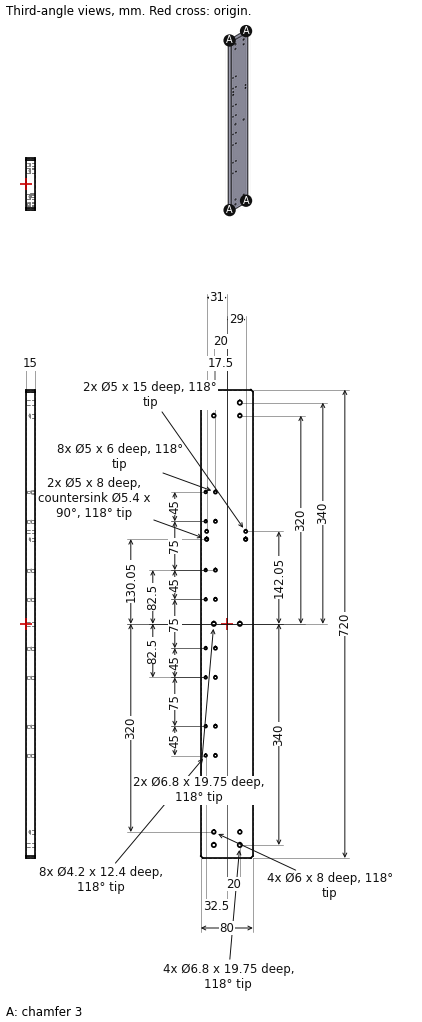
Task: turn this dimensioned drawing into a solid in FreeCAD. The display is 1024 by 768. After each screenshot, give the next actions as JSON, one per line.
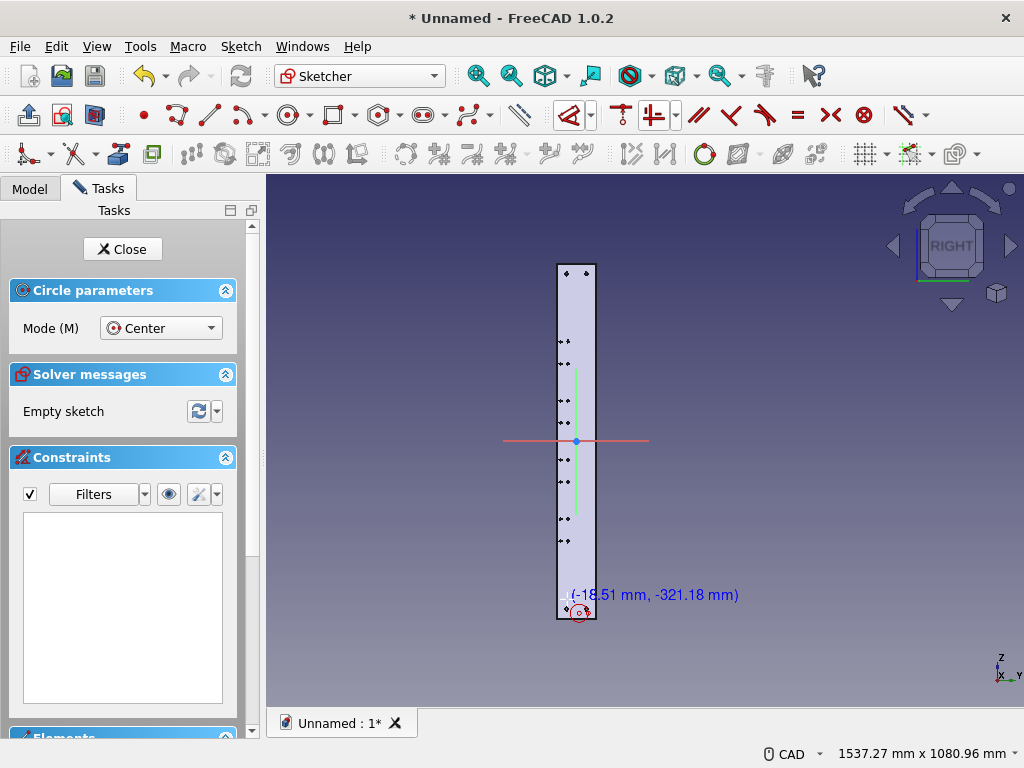
{"action": "scroll", "coordinate": [567, 599], "scroll_direction": "up", "scroll_amount": 3}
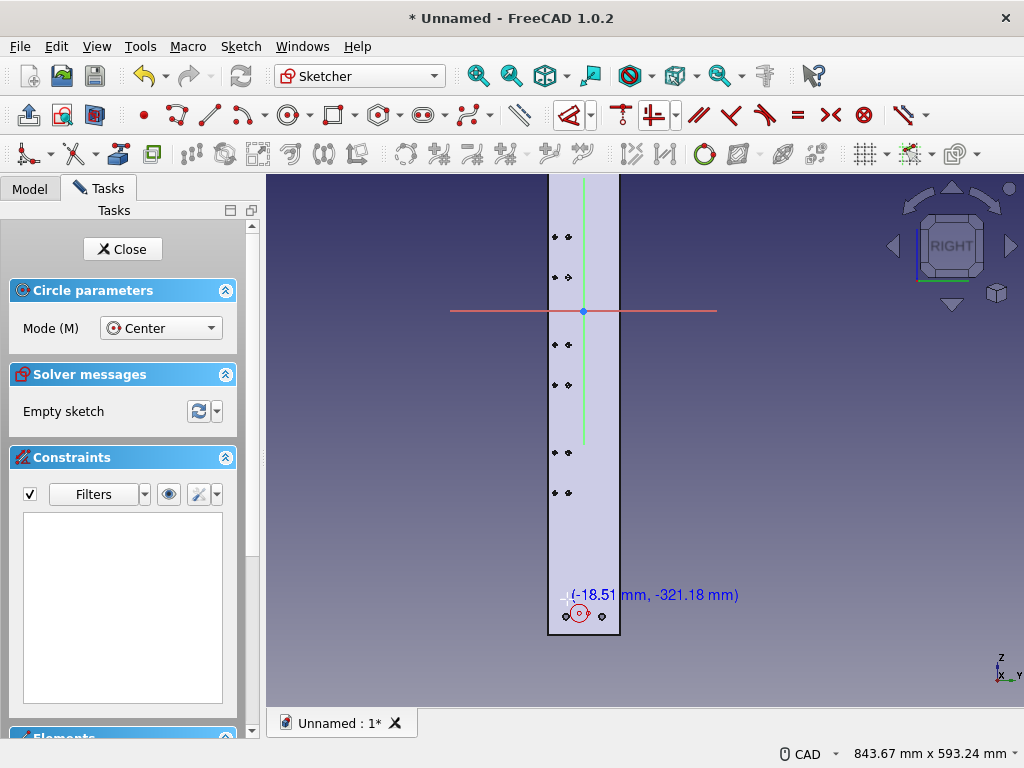
{"action": "left_click", "coordinate": [566, 599]}
{"action": "mouse_move", "coordinate": [568, 597]}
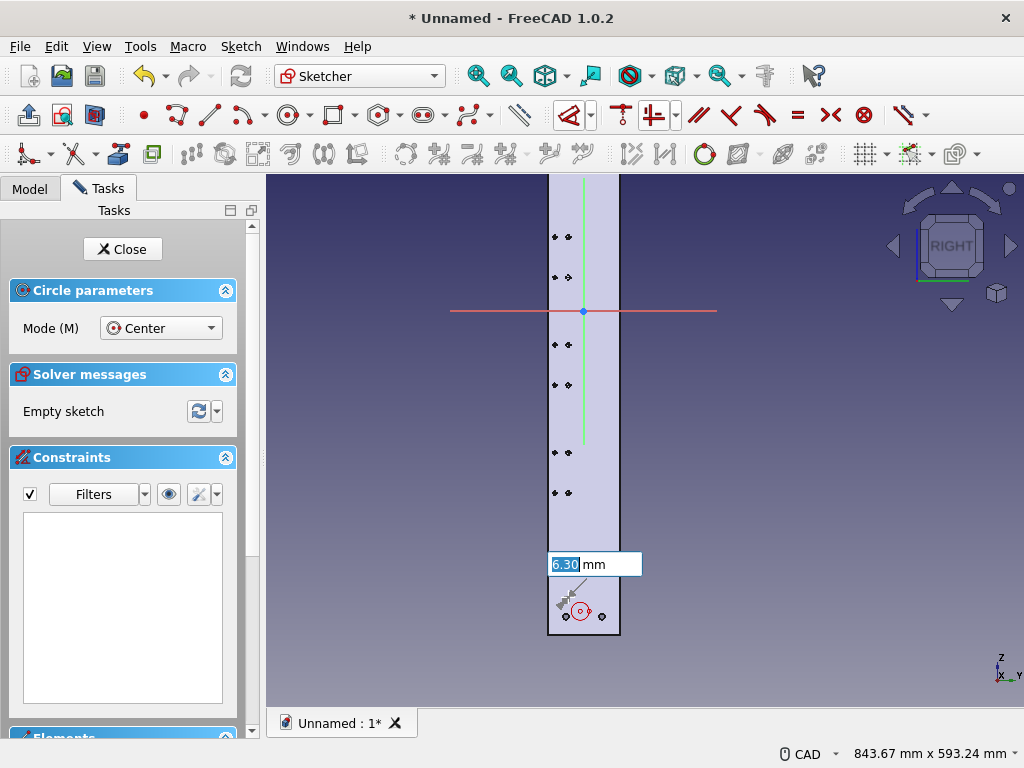
{"action": "type", "text": "6"}
{"action": "key", "text": "Return"}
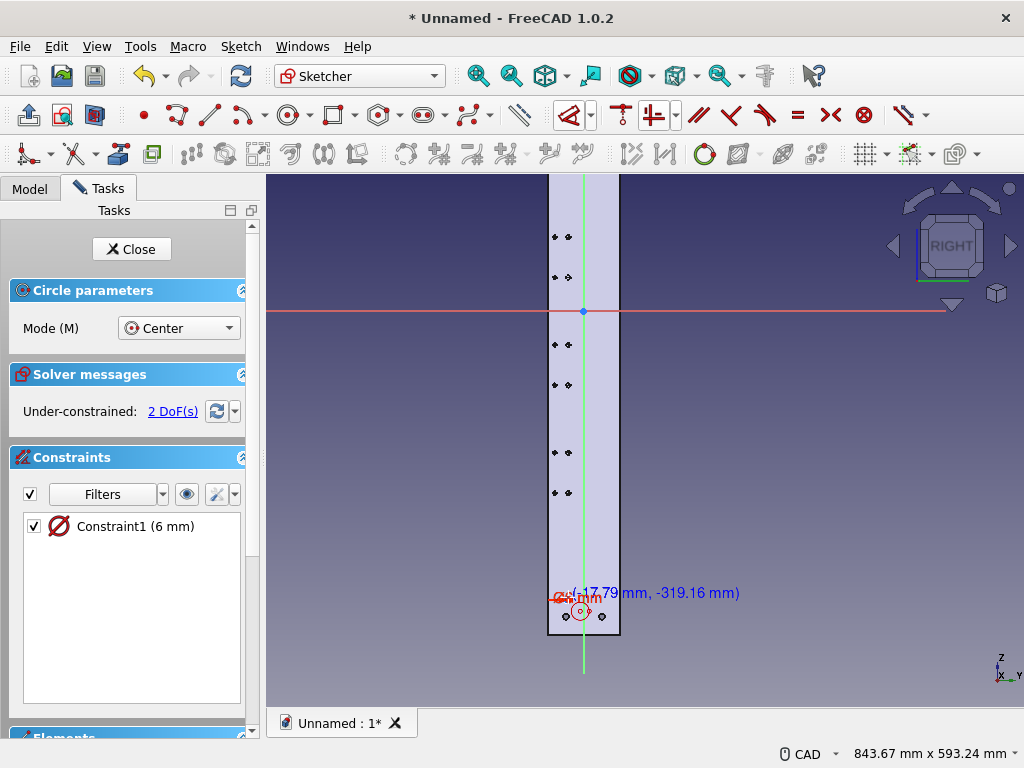
{"action": "scroll", "coordinate": [567, 598], "scroll_direction": "down", "scroll_amount": 3}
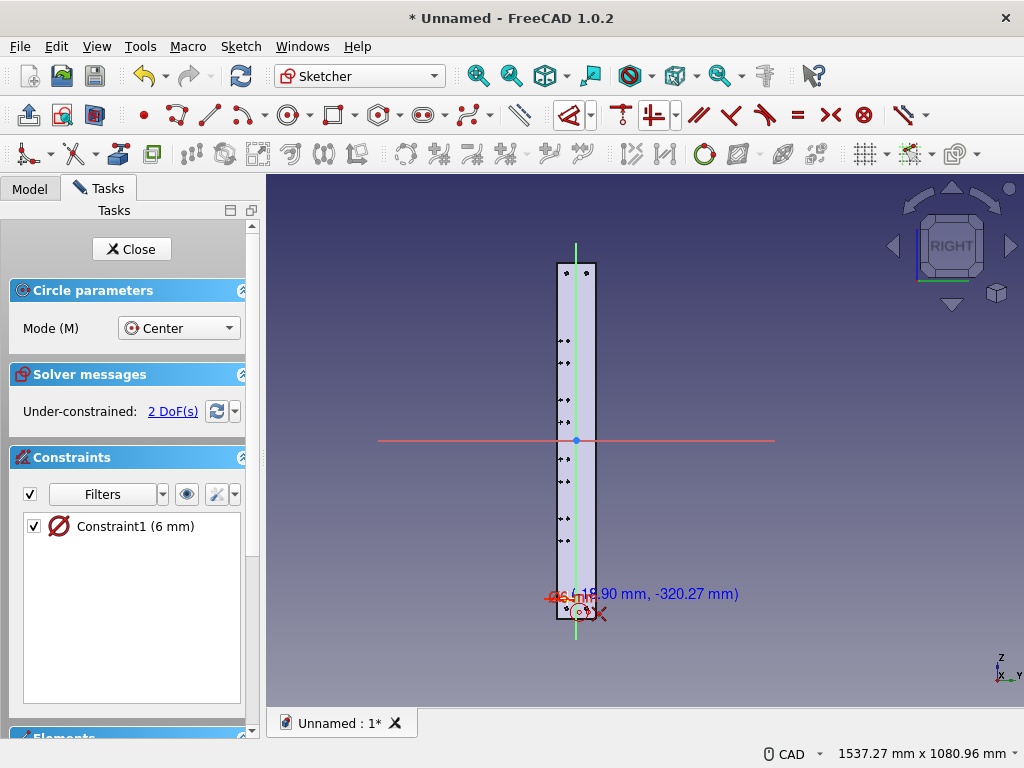
{"action": "scroll", "coordinate": [586, 283], "scroll_direction": "up", "scroll_amount": 14}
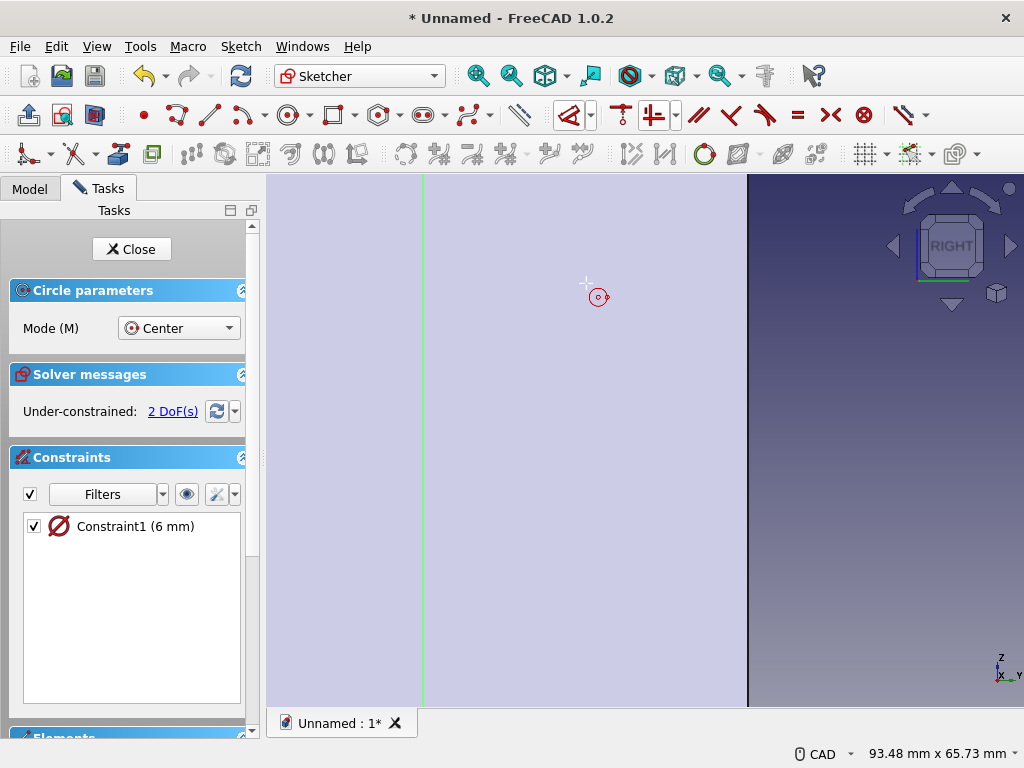
{"action": "scroll", "coordinate": [586, 283], "scroll_direction": "down", "scroll_amount": 14}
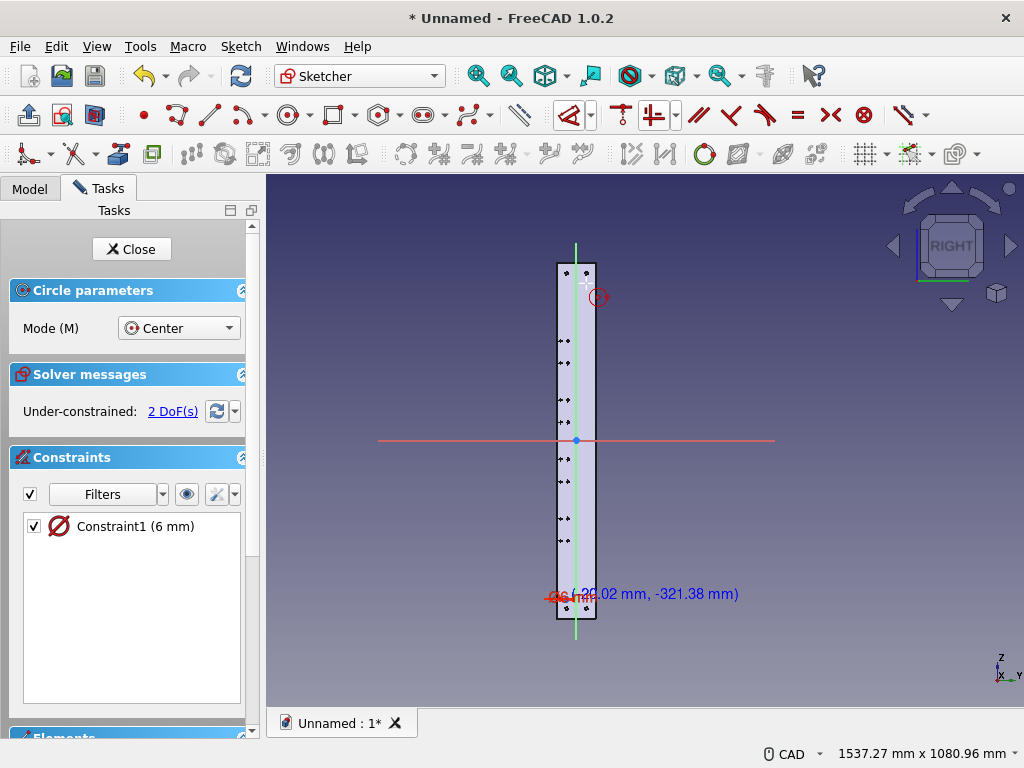
{"action": "scroll", "coordinate": [586, 283], "scroll_direction": "up", "scroll_amount": 3}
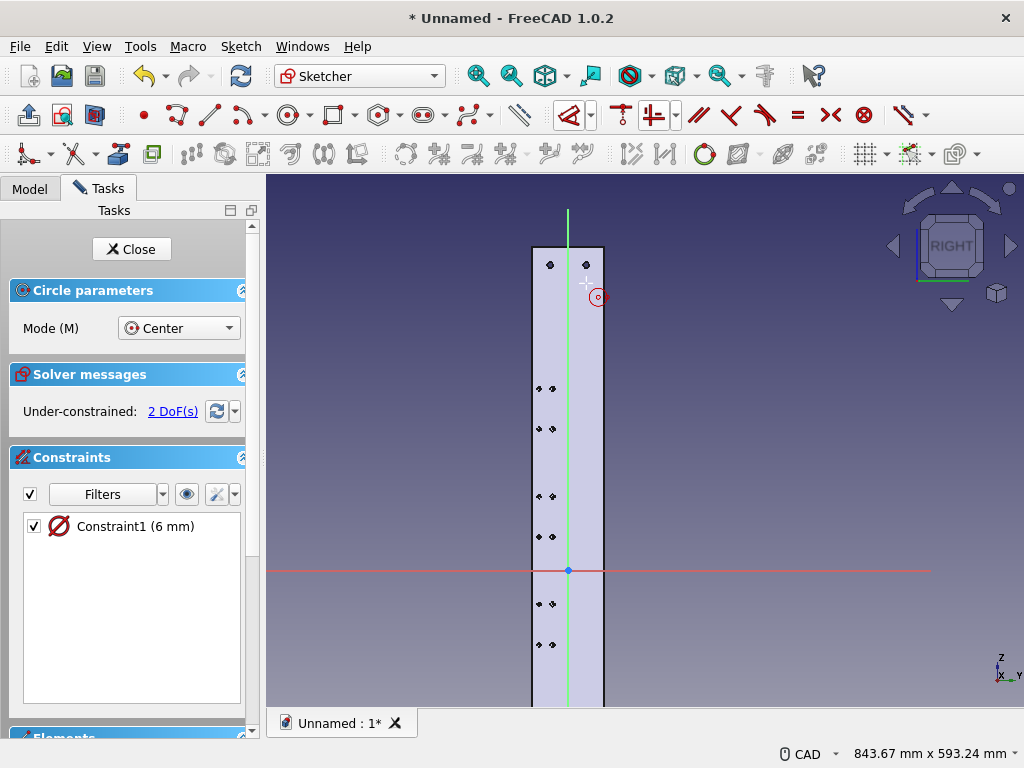
{"action": "left_click", "coordinate": [586, 283]}
{"action": "mouse_move", "coordinate": [588, 281]}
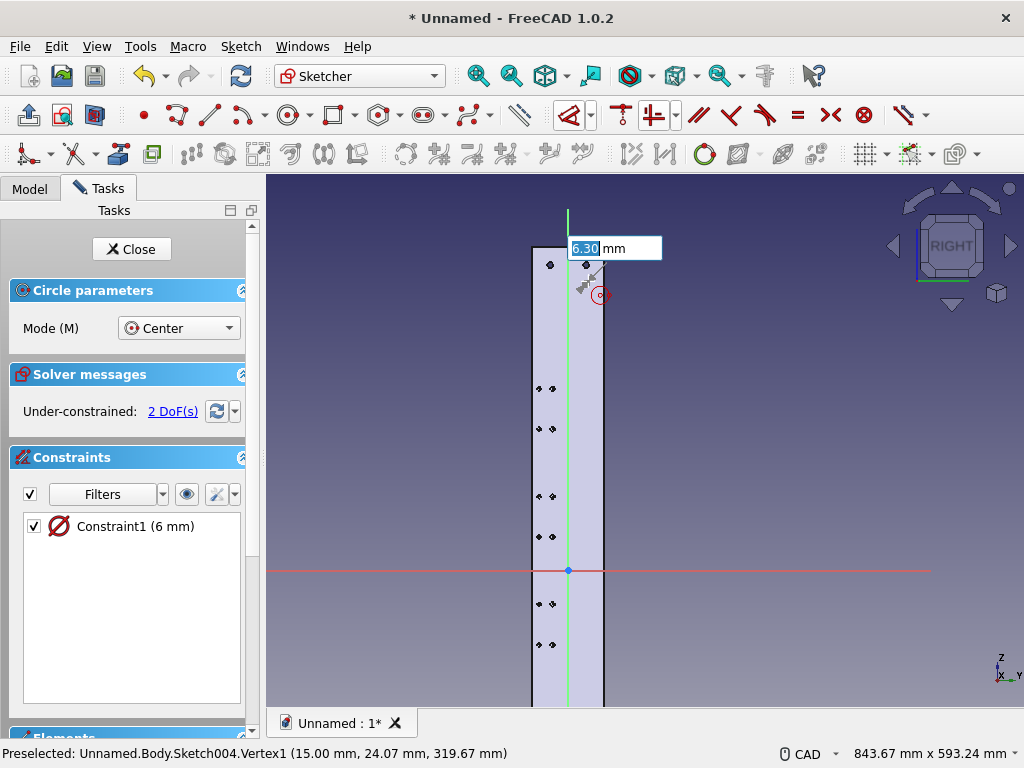
{"action": "type", "text": "6"}
{"action": "key", "text": "Return"}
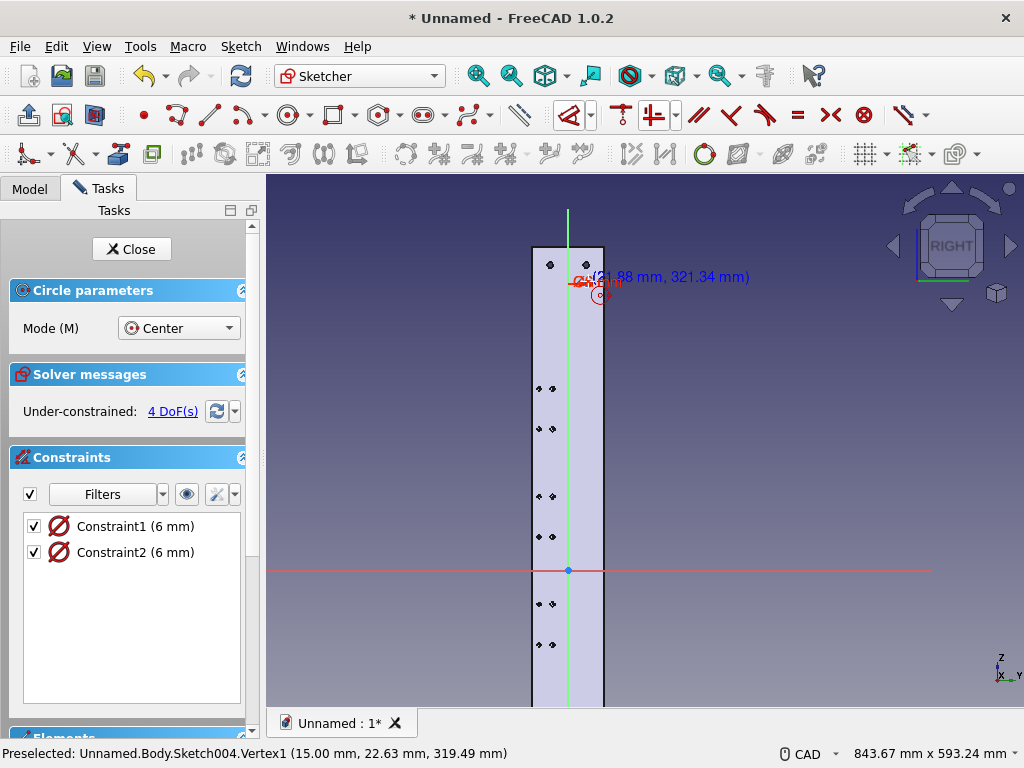
{"action": "scroll", "coordinate": [550, 283], "scroll_direction": "up", "scroll_amount": 11}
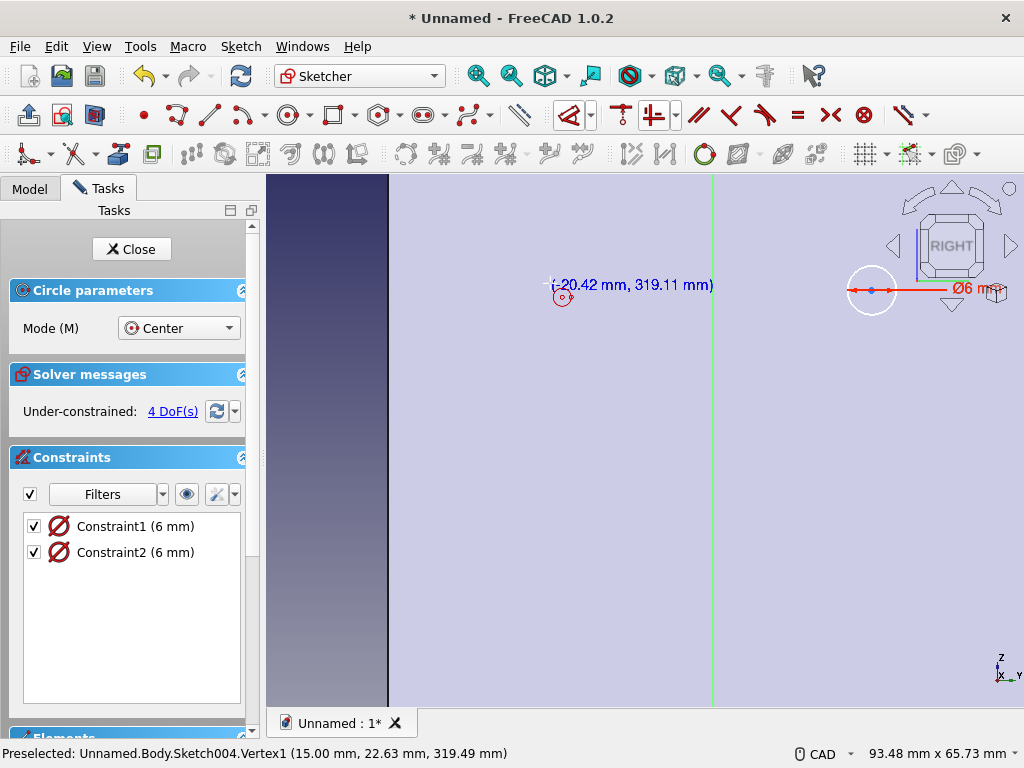
{"action": "scroll", "coordinate": [568, 283], "scroll_direction": "down", "scroll_amount": 14}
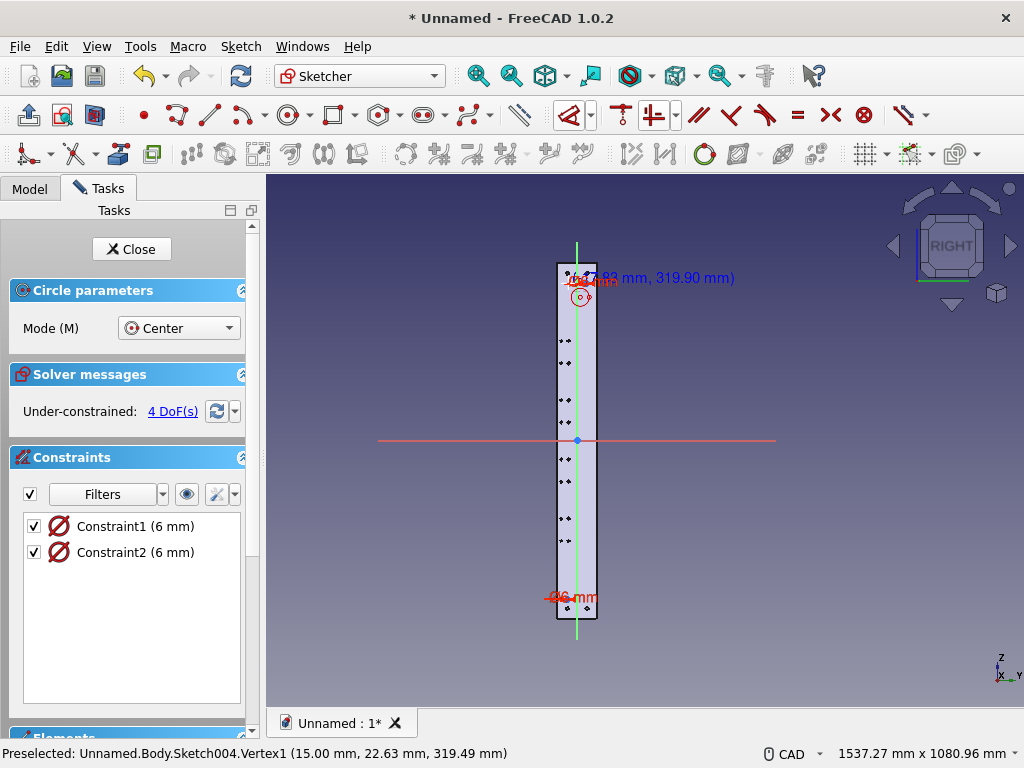
{"action": "scroll", "coordinate": [567, 283], "scroll_direction": "up", "scroll_amount": 3}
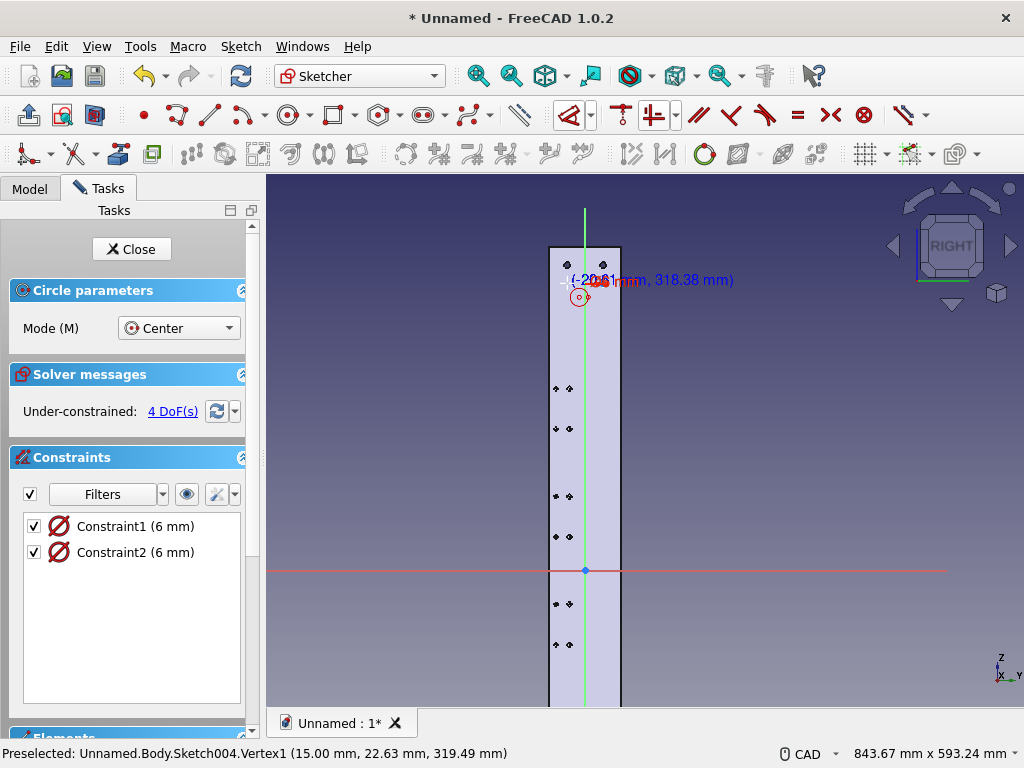
{"action": "left_click", "coordinate": [567, 283]}
{"action": "mouse_move", "coordinate": [569, 281]}